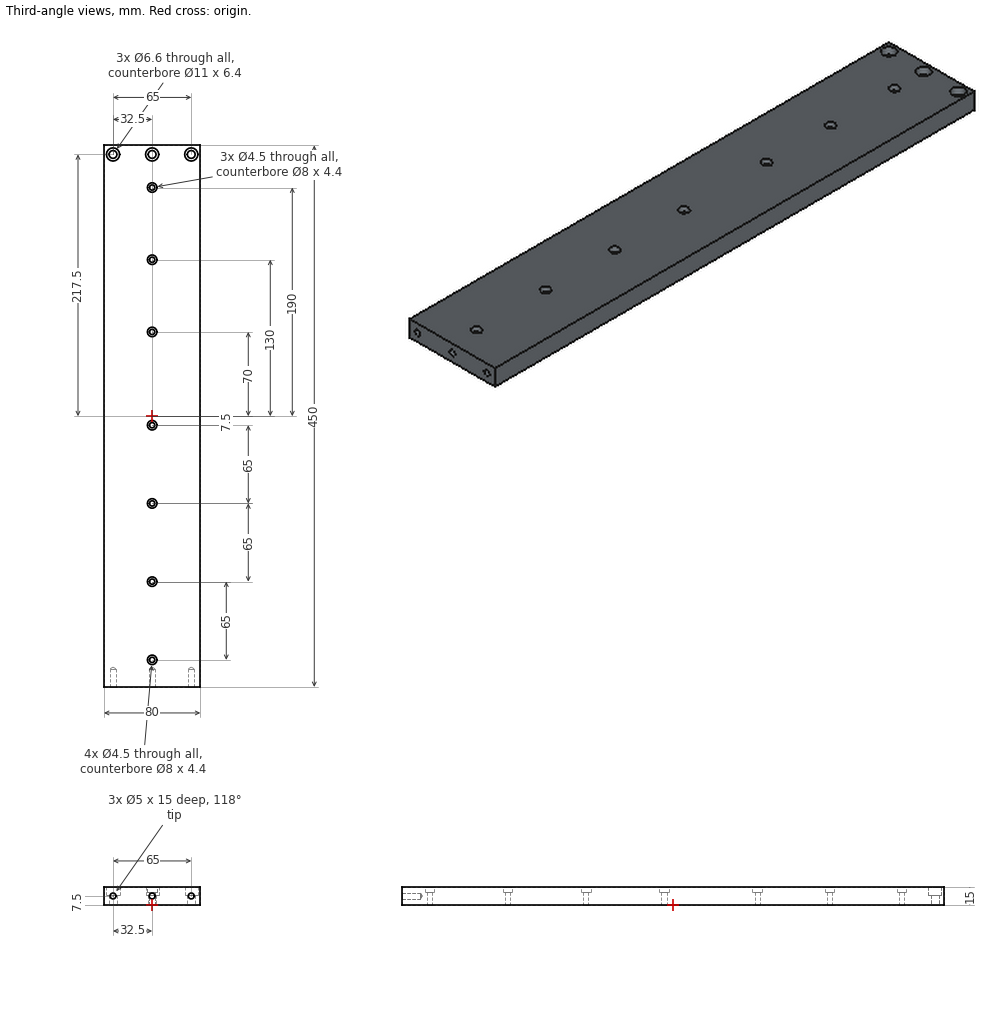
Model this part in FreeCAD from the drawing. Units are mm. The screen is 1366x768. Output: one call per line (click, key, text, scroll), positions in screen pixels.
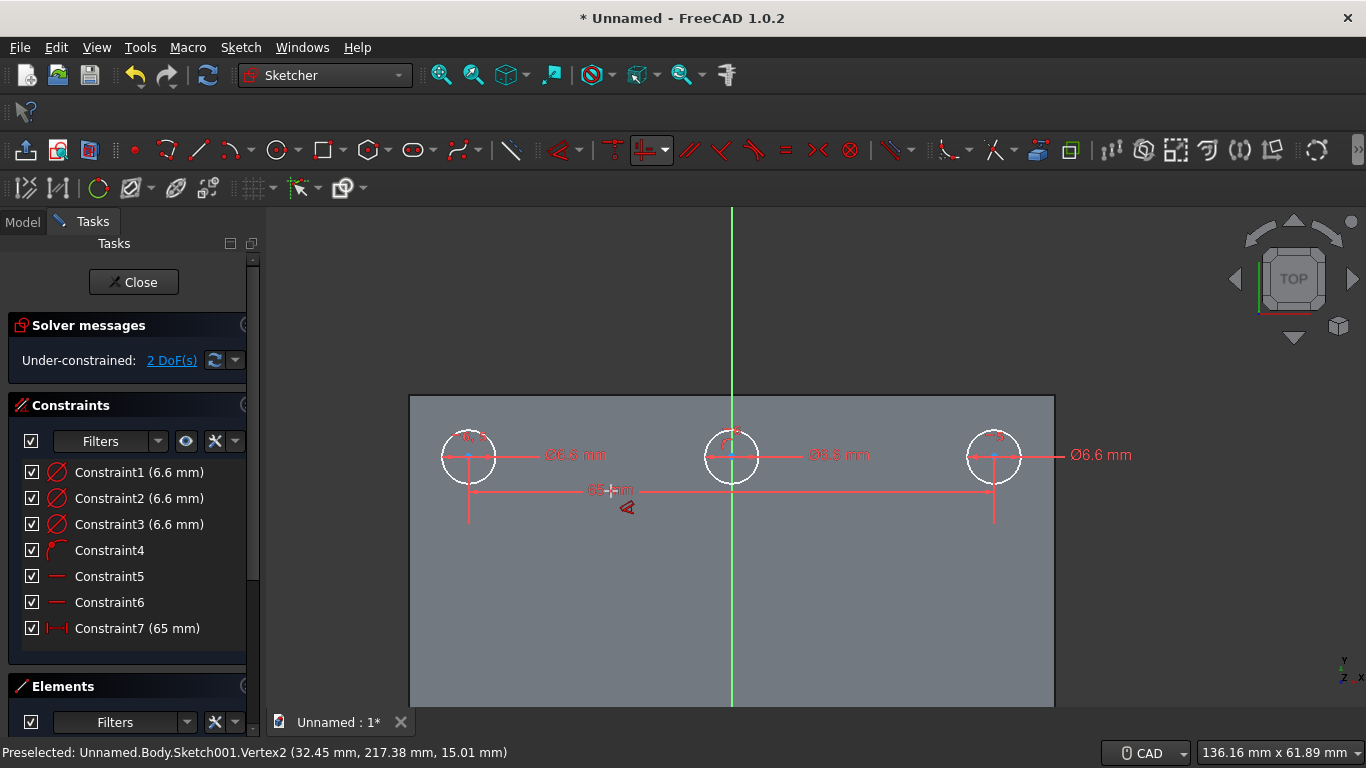
click(469, 457)
click(600, 423)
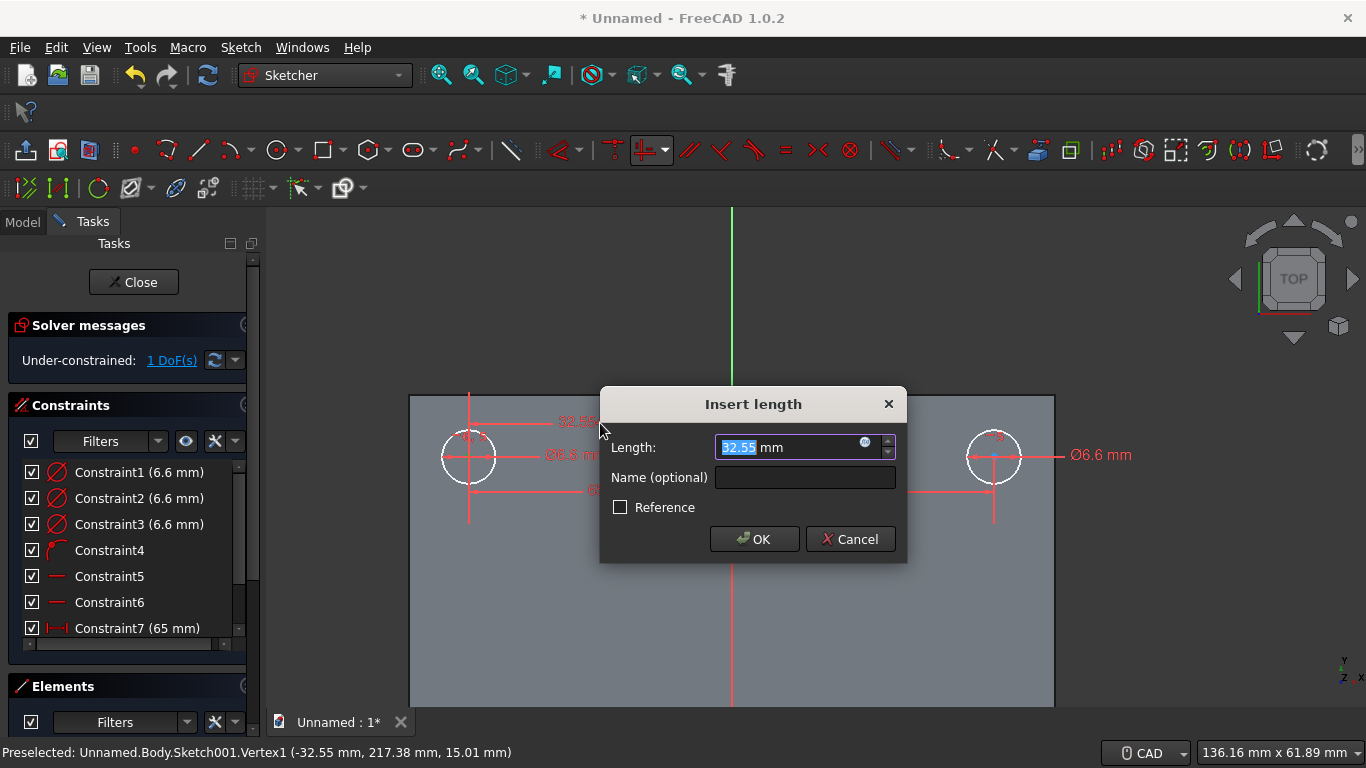
text(32.5)
key(Return)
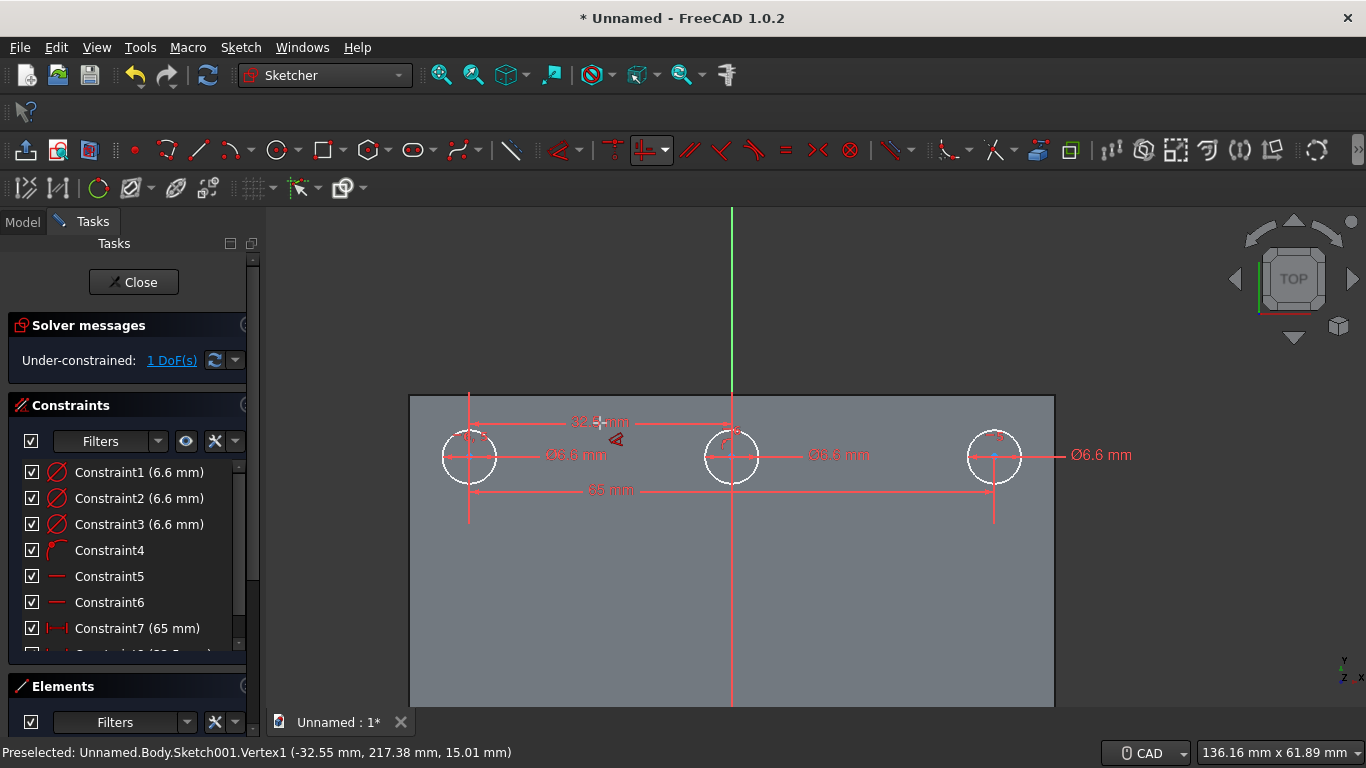
click(469, 457)
click(435, 568)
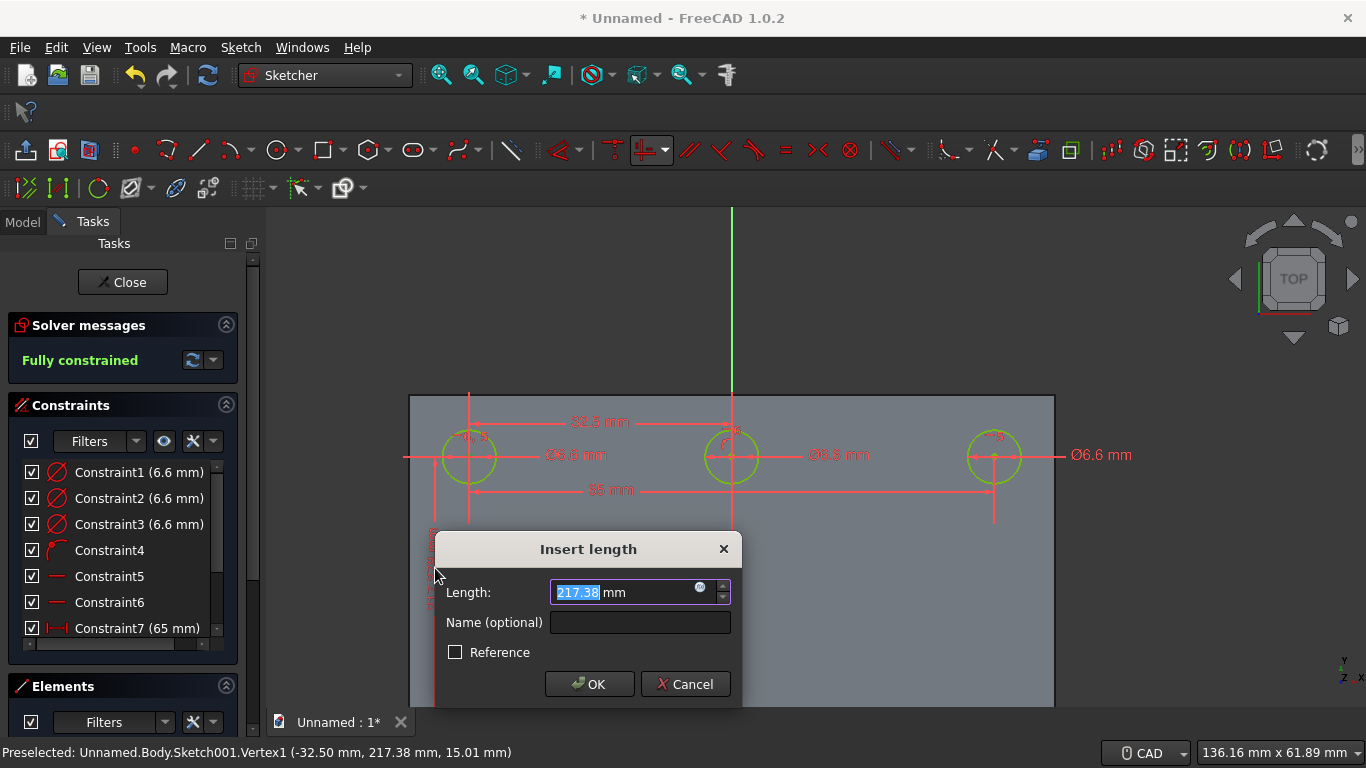
text(217.5)
key(Return)
key(Escape)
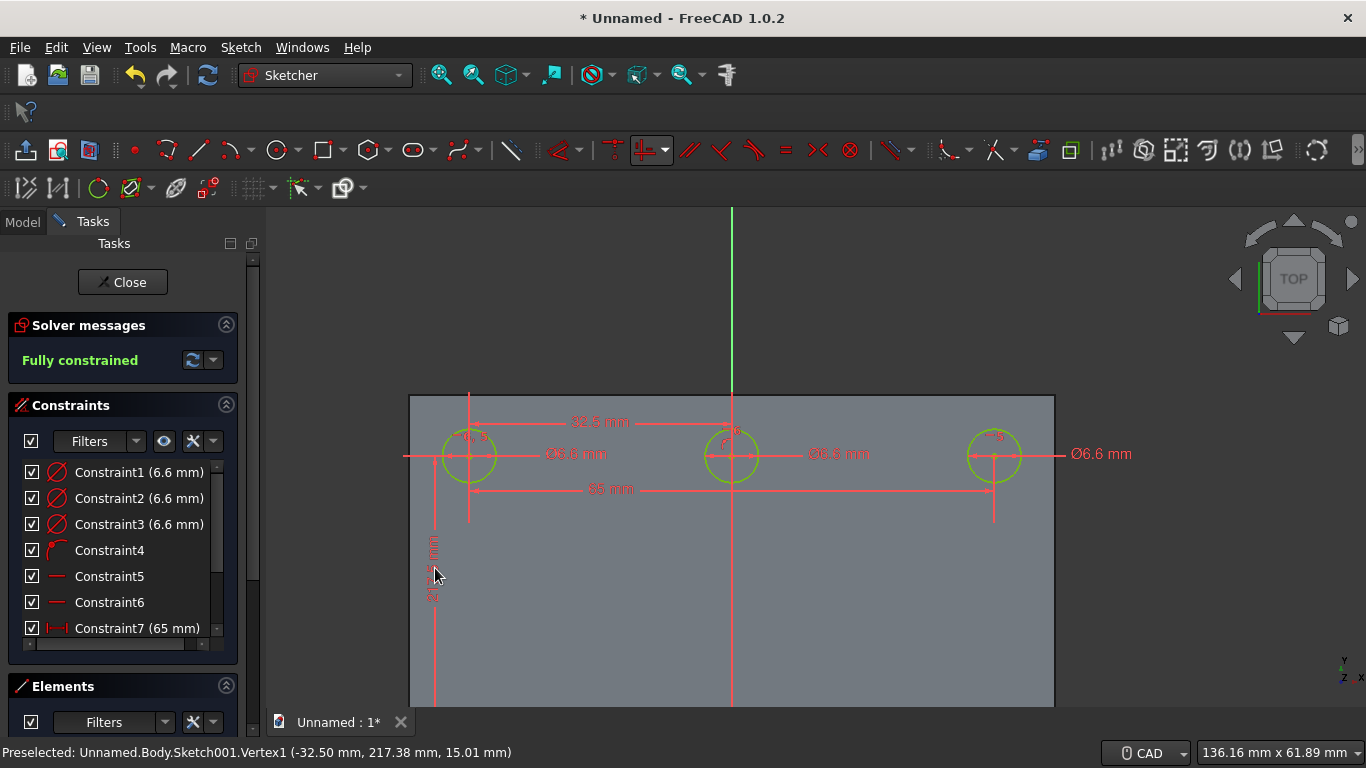
click(123, 282)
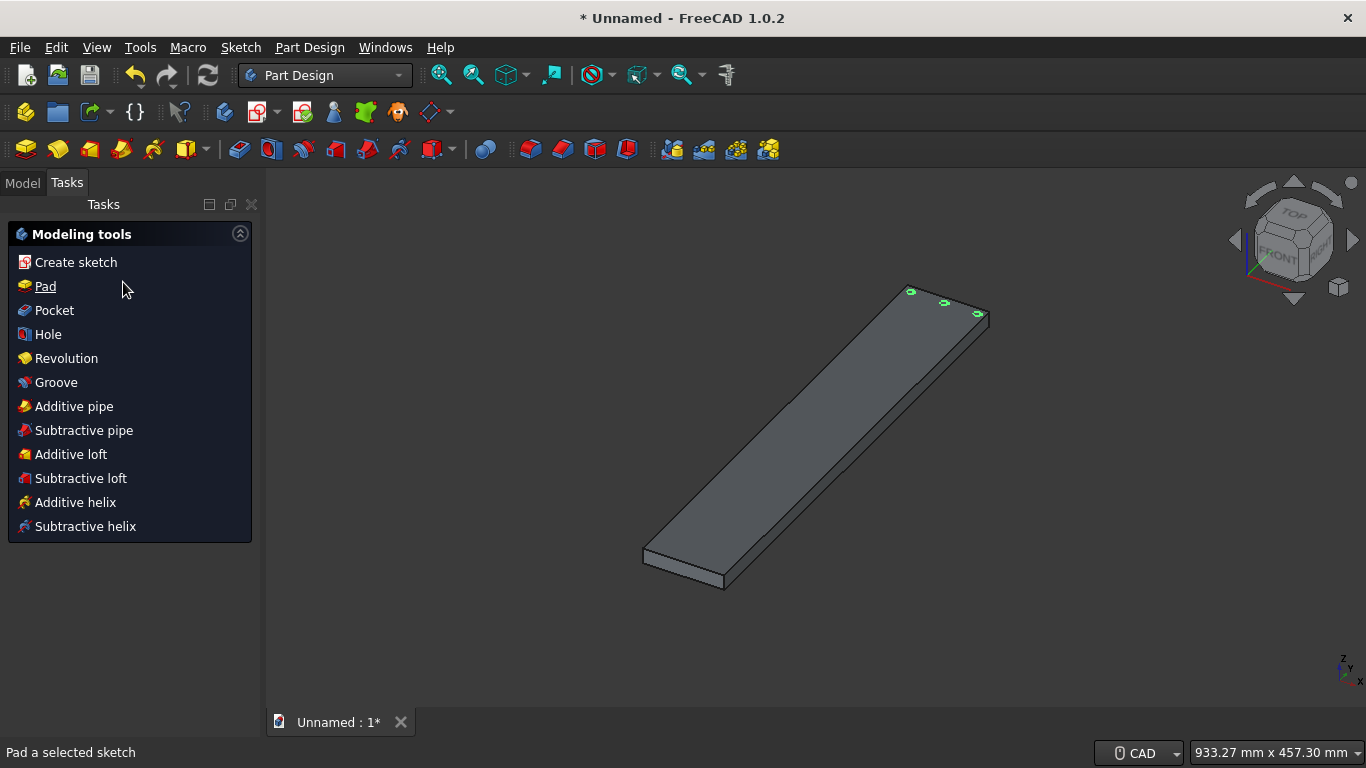
click(272, 150)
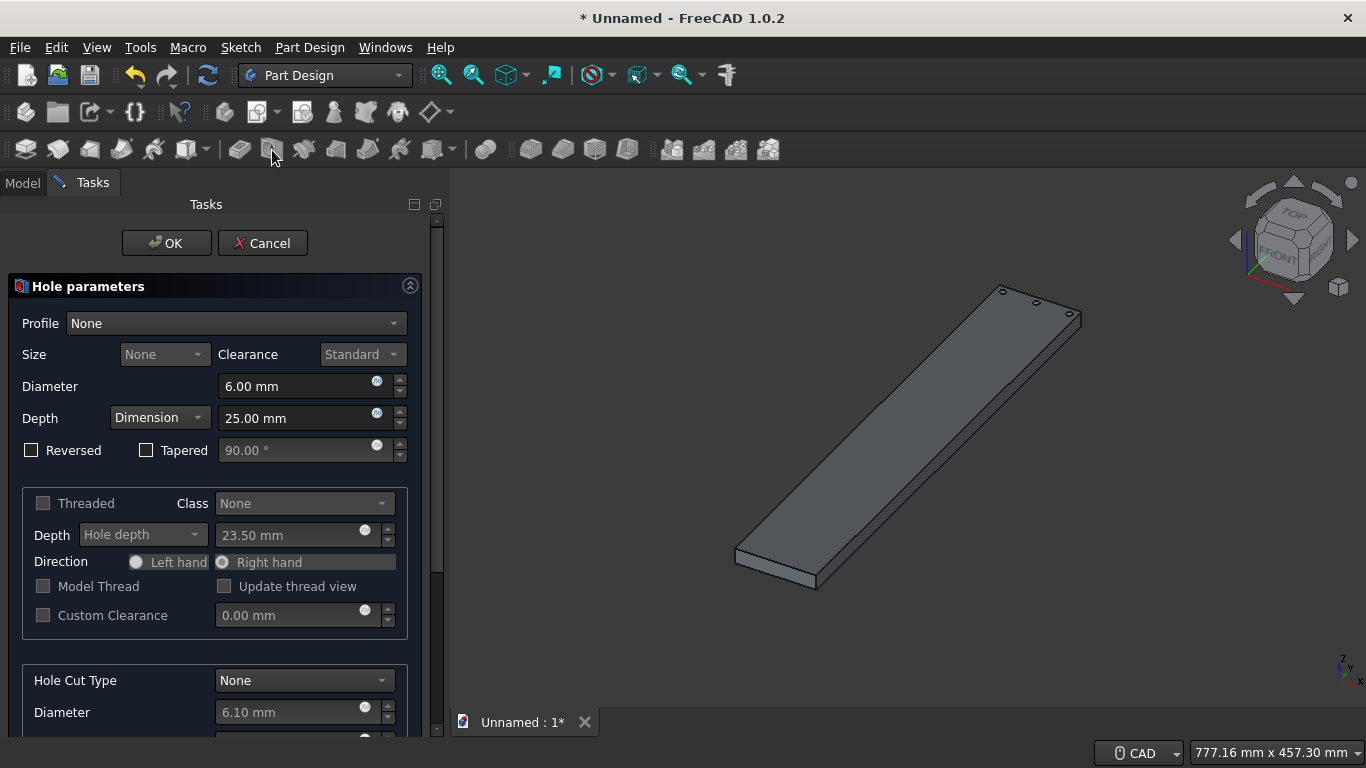
triple_click(305, 386)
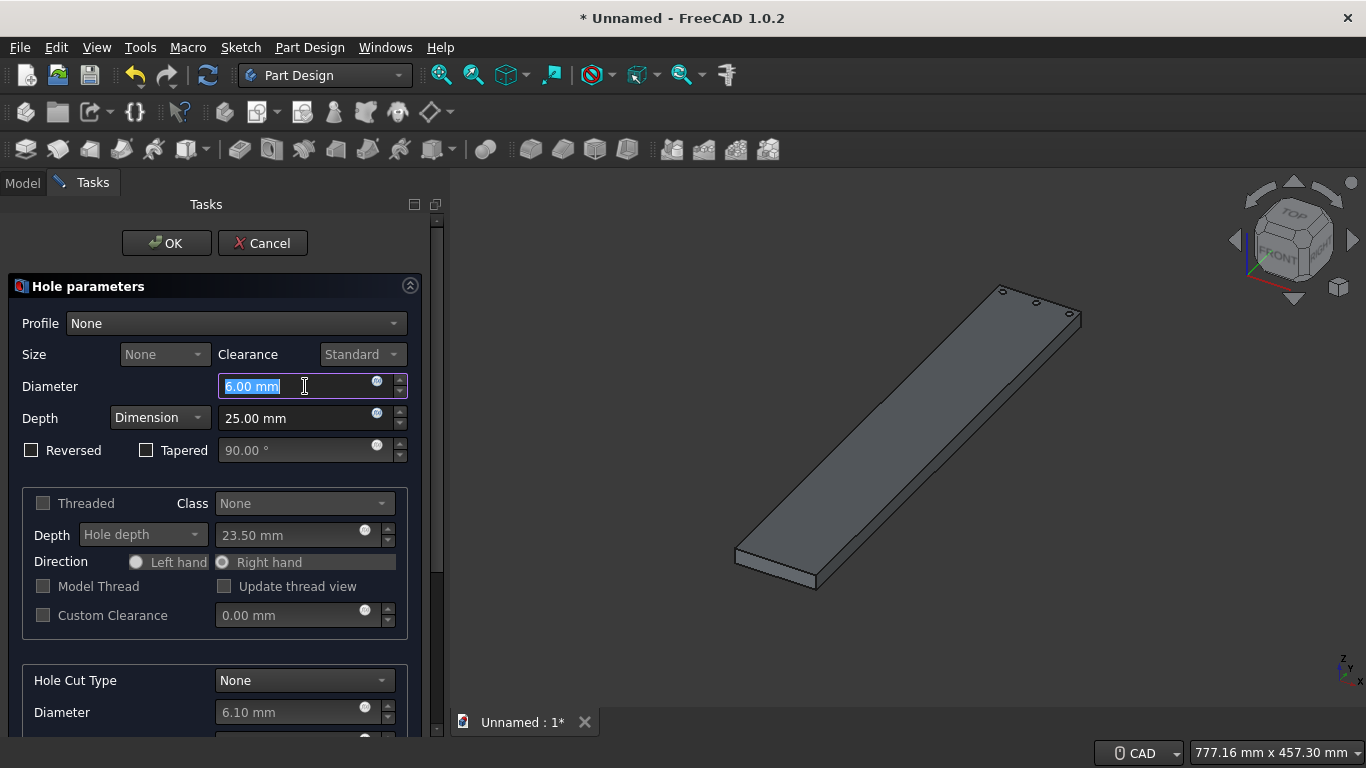
text(6.6)
key(Tab)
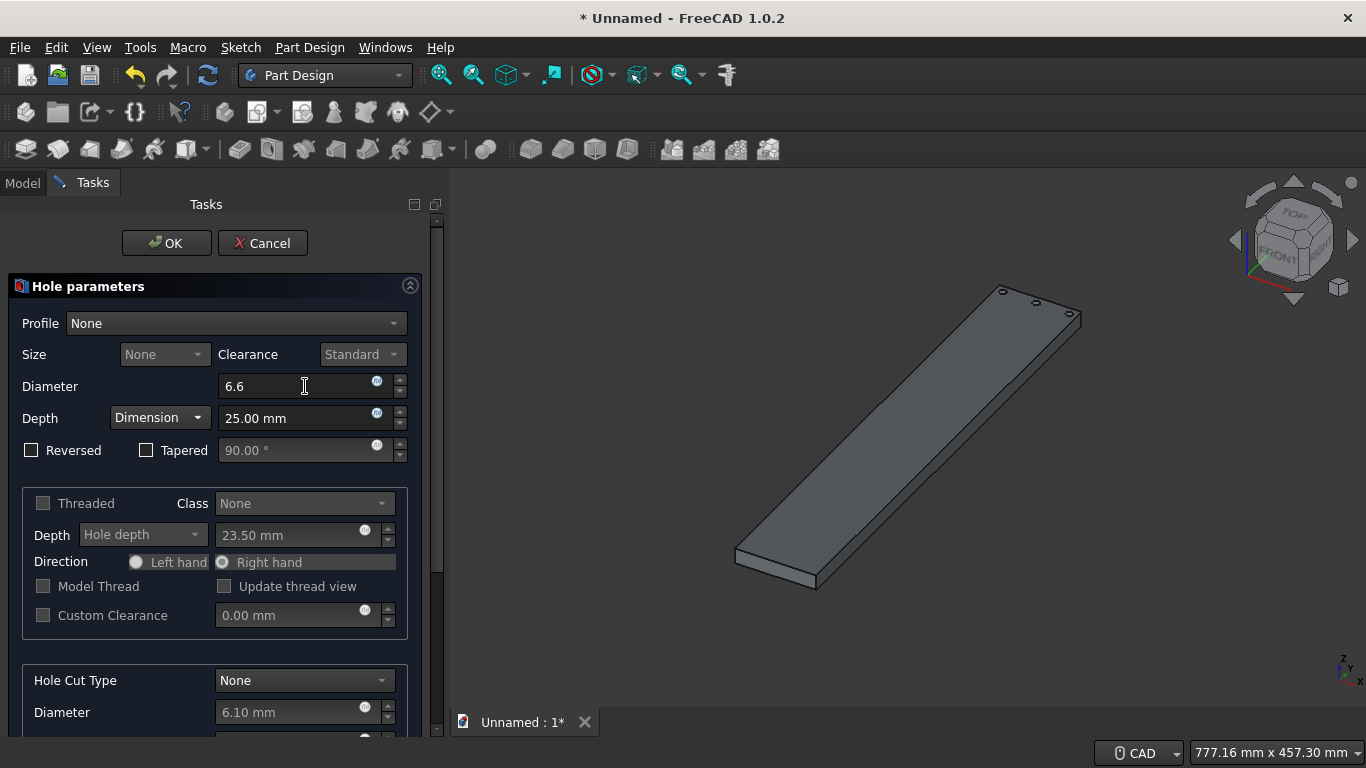
click(161, 418)